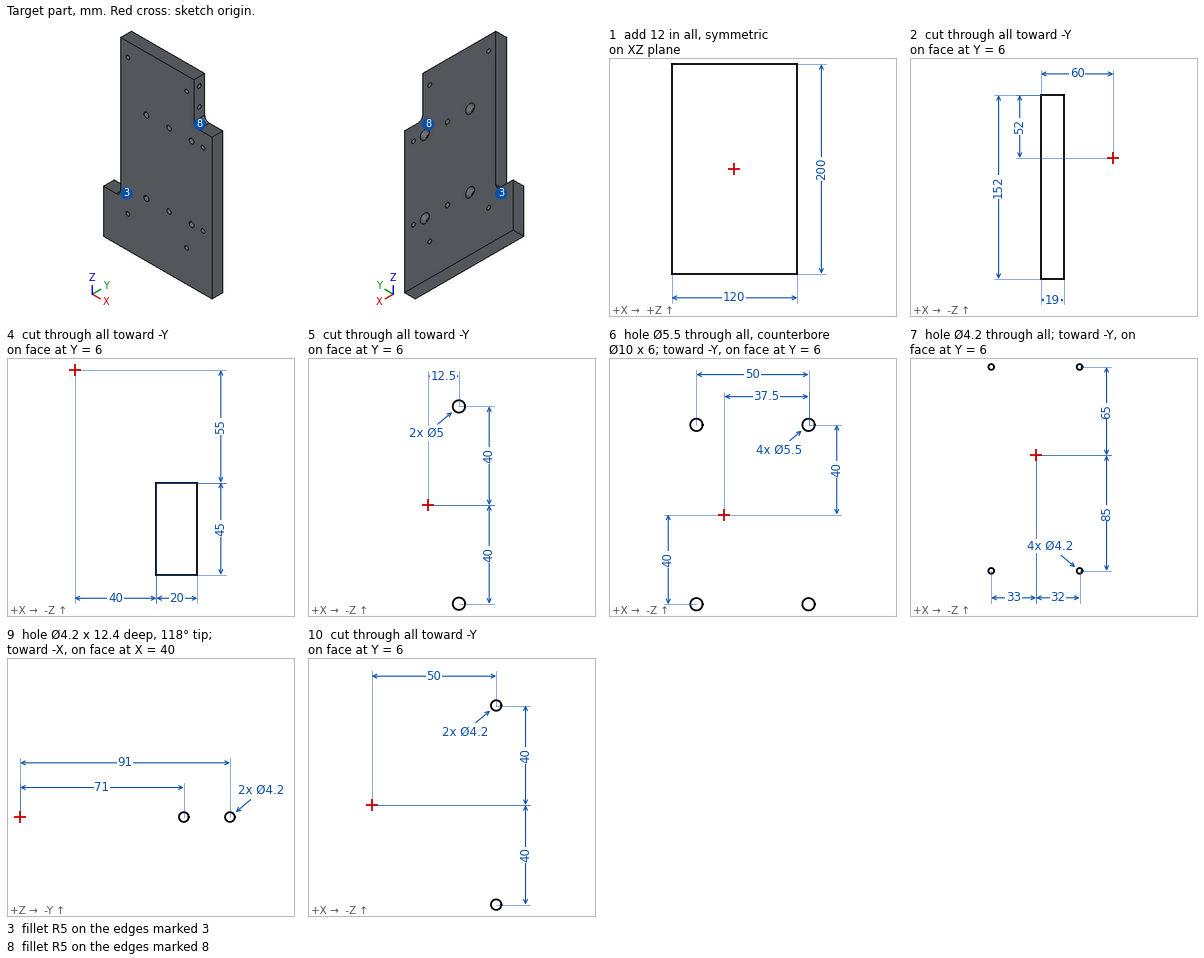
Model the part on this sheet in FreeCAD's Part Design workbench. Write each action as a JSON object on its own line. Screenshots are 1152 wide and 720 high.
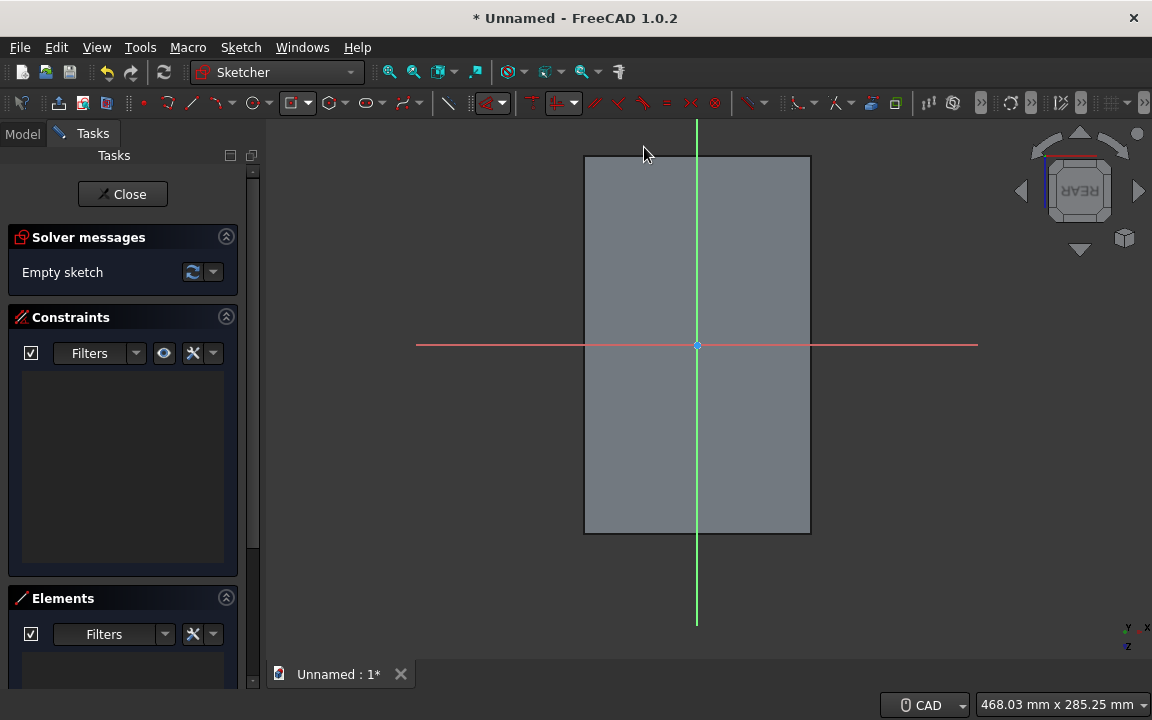
{"action": "left_click", "coordinate": [310, 104]}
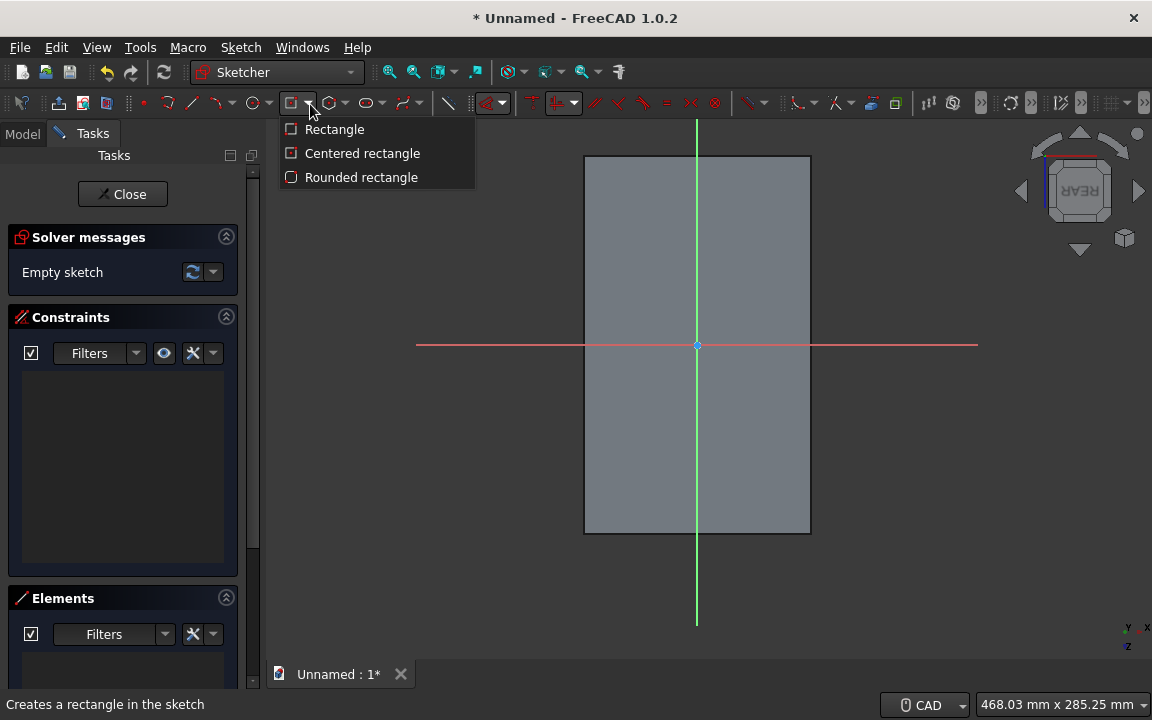
{"action": "left_click", "coordinate": [378, 129]}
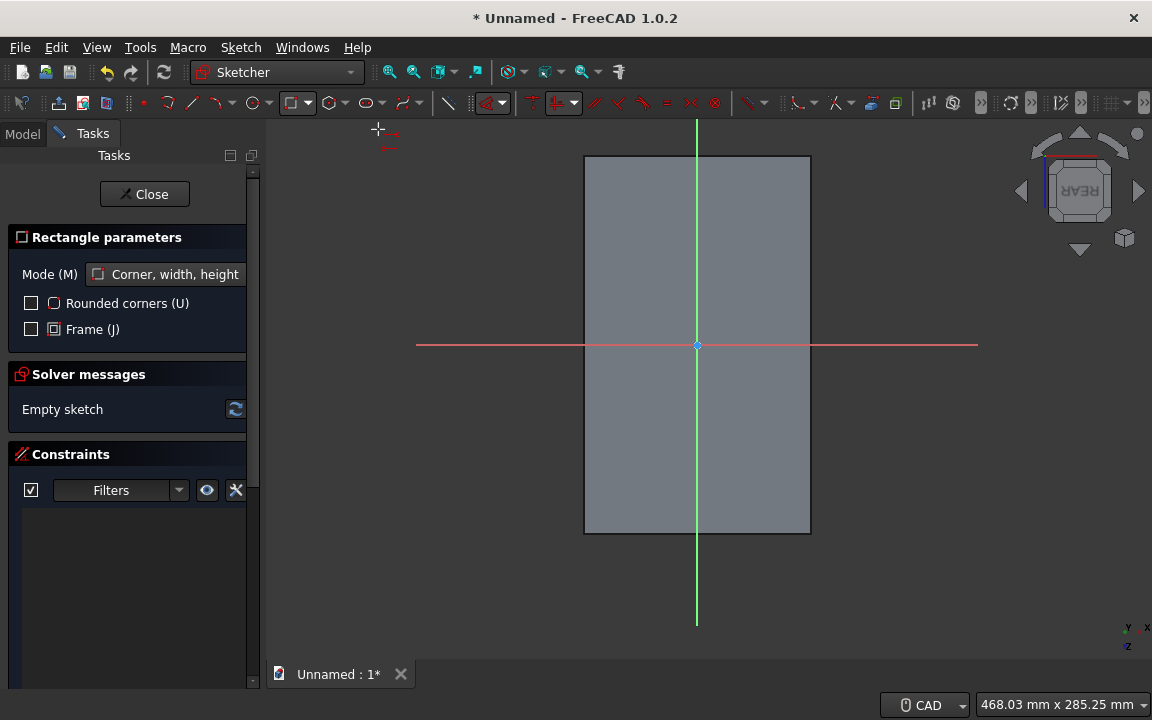
{"action": "left_click", "coordinate": [584, 247]}
{"action": "left_click", "coordinate": [620, 534]}
{"action": "key", "text": "Escape"}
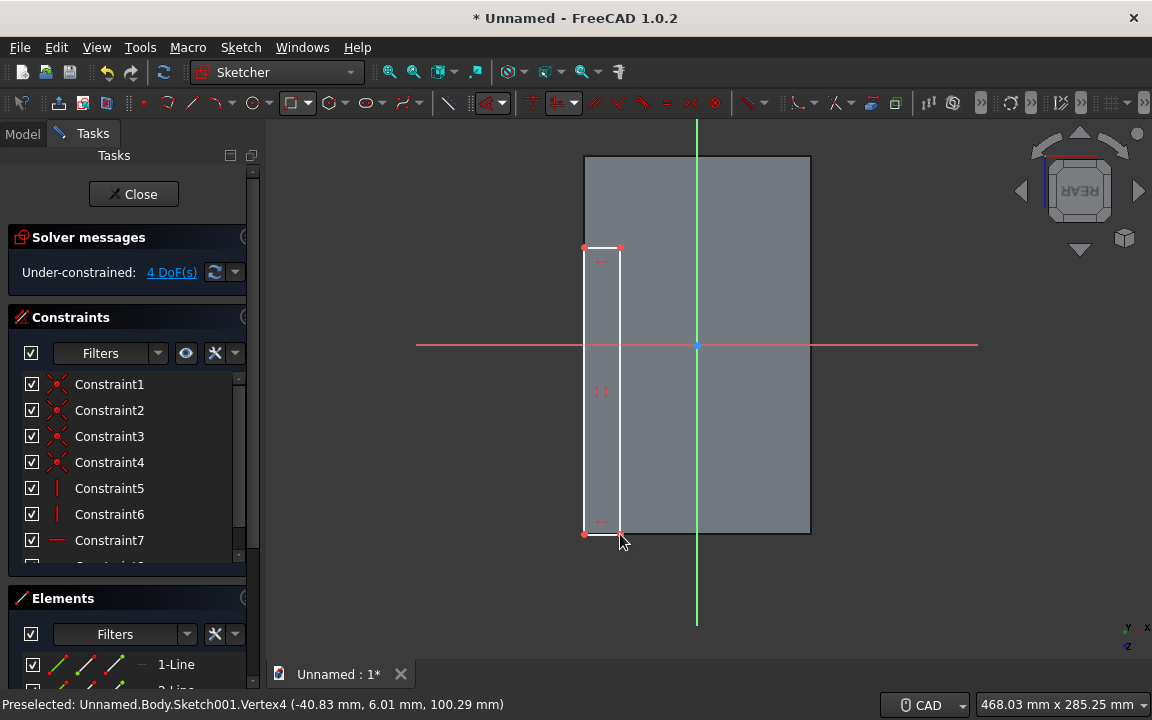
{"action": "scroll", "coordinate": [595, 535], "scroll_direction": "up", "scroll_amount": 2}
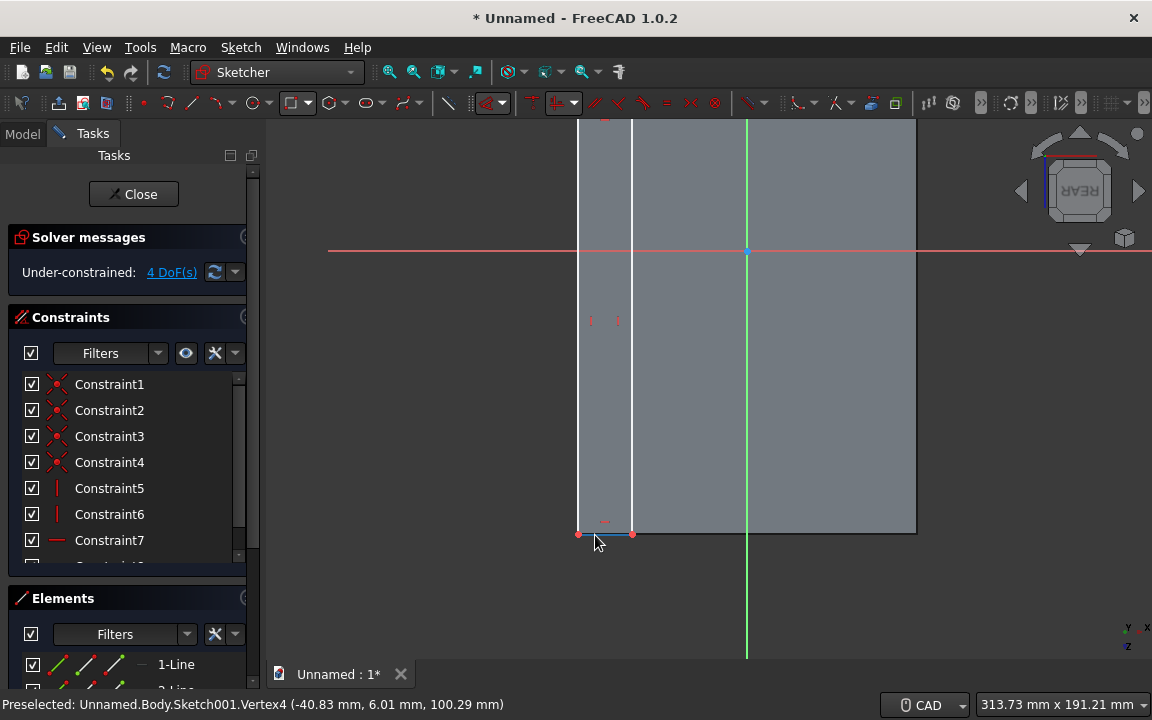
{"action": "left_click", "coordinate": [595, 535]}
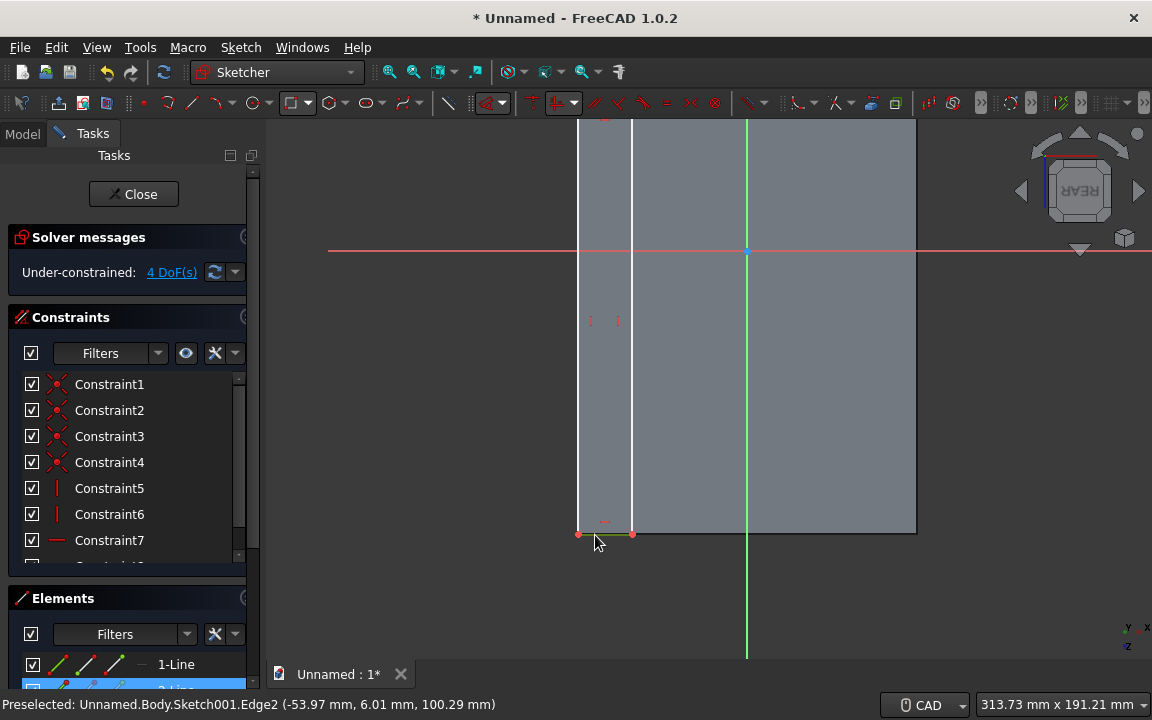
{"action": "left_click", "coordinate": [504, 104]}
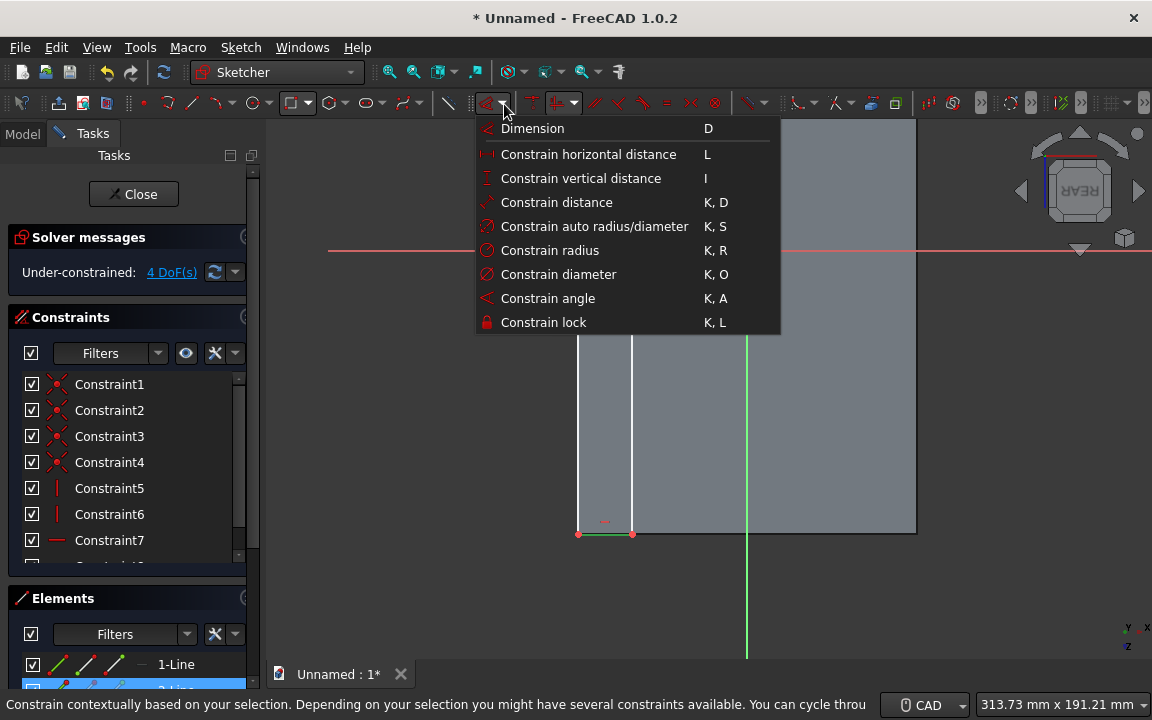
{"action": "left_click", "coordinate": [628, 154]}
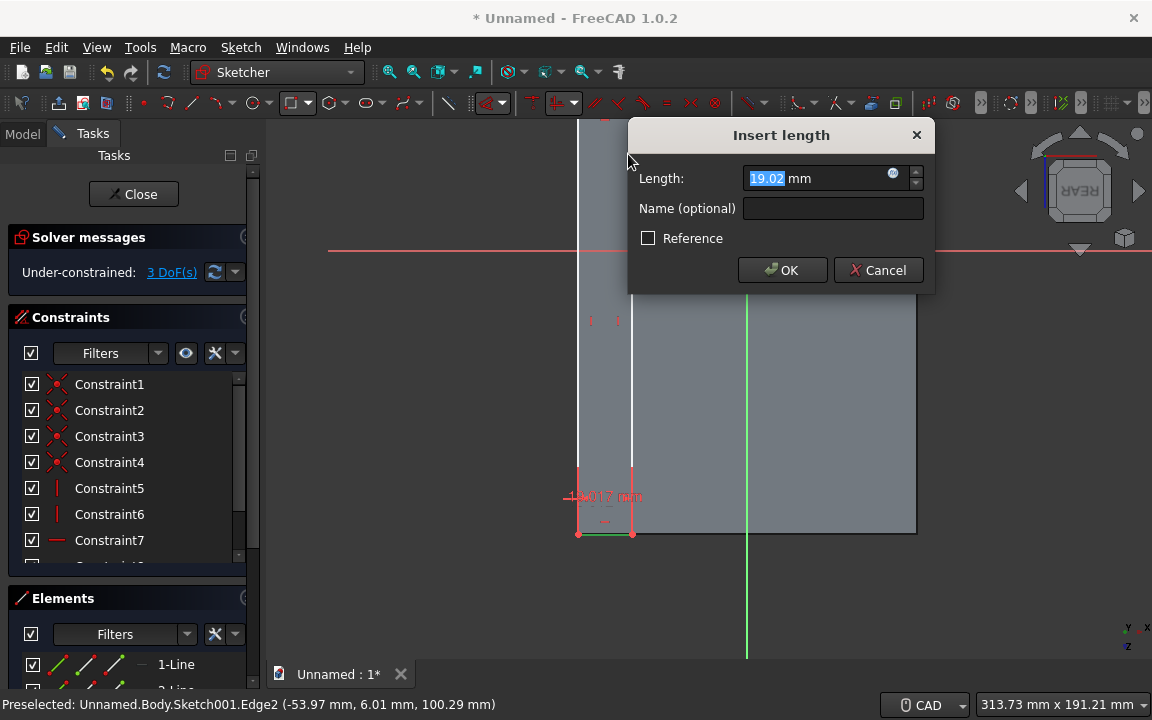
{"action": "type", "text": "19"}
{"action": "key", "text": "Return"}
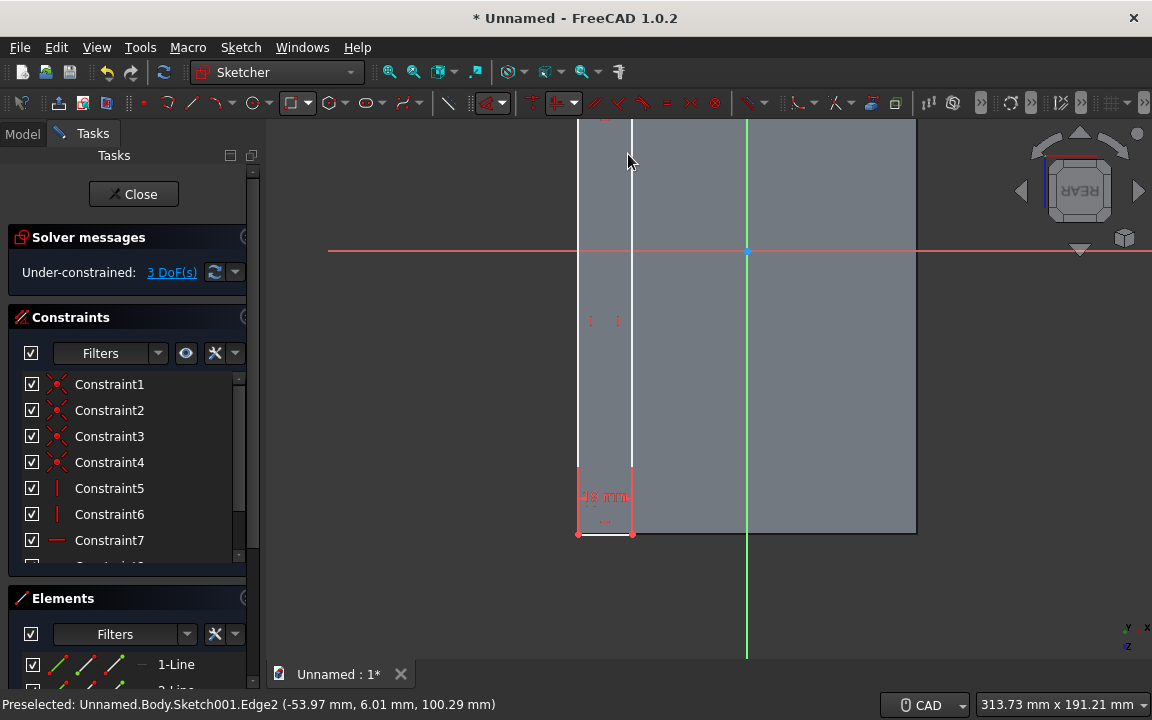
{"action": "left_click", "coordinate": [578, 235]}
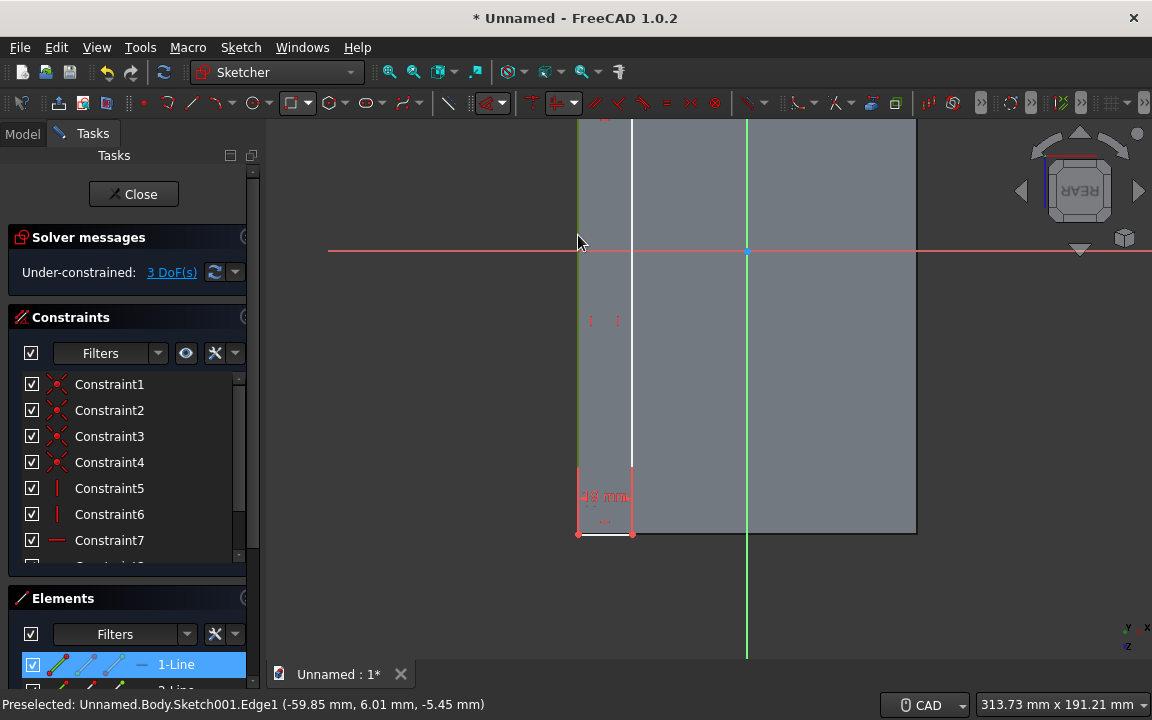
{"action": "key", "text": "i"}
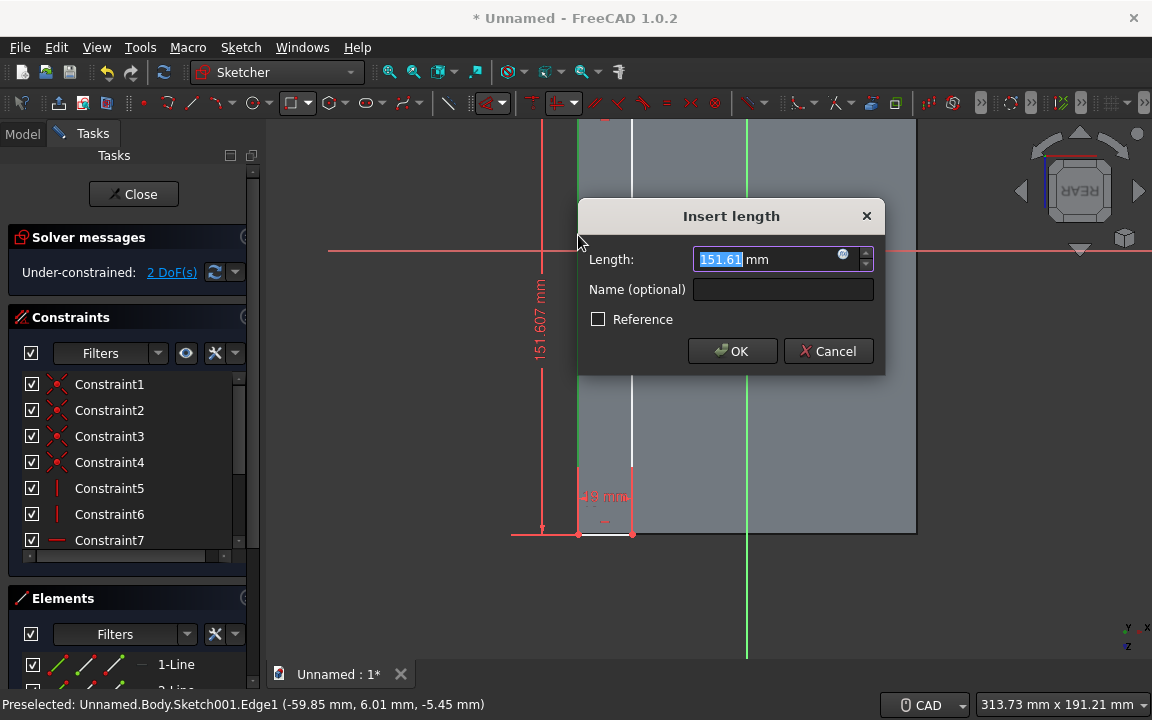
{"action": "type", "text": "152"}
{"action": "key", "text": "Return"}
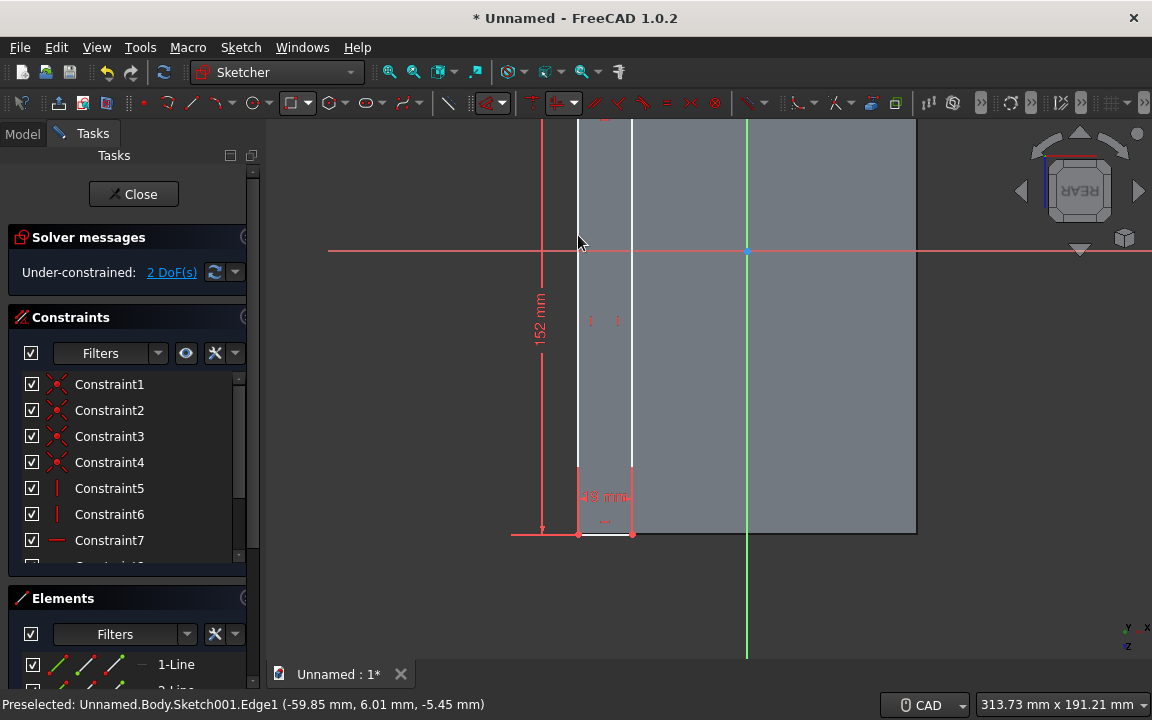
{"action": "scroll", "coordinate": [540, 631], "scroll_direction": "down", "scroll_amount": 1}